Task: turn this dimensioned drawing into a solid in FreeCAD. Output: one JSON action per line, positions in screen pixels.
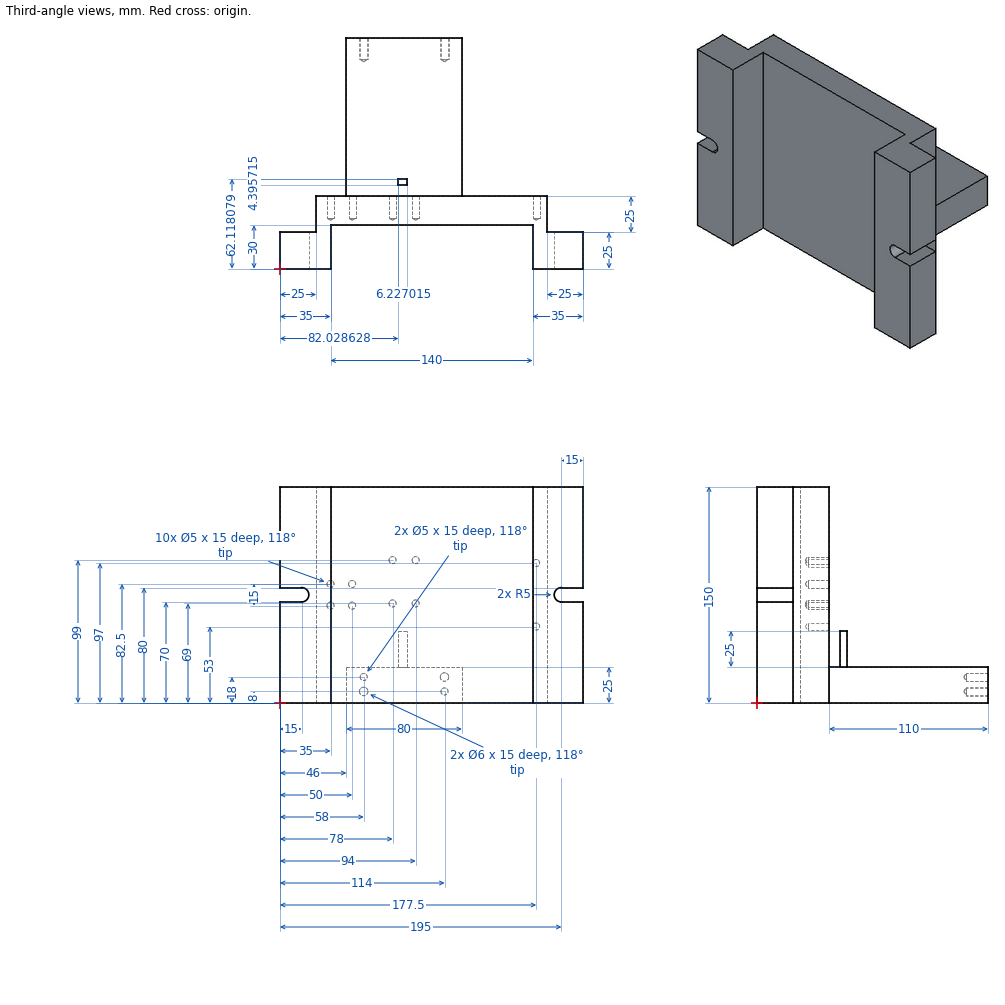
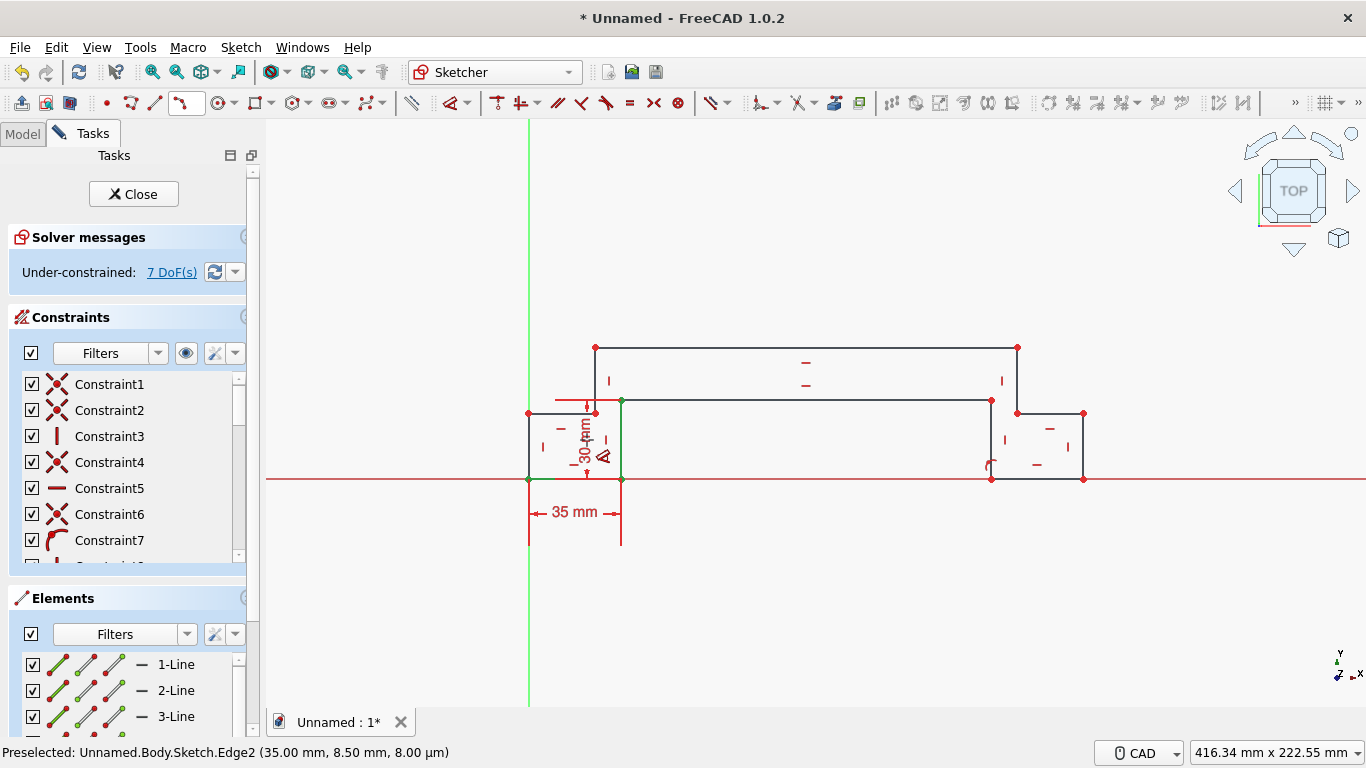
{"action": "left_click", "coordinate": [1019, 479]}
{"action": "left_click", "coordinate": [1037, 513]}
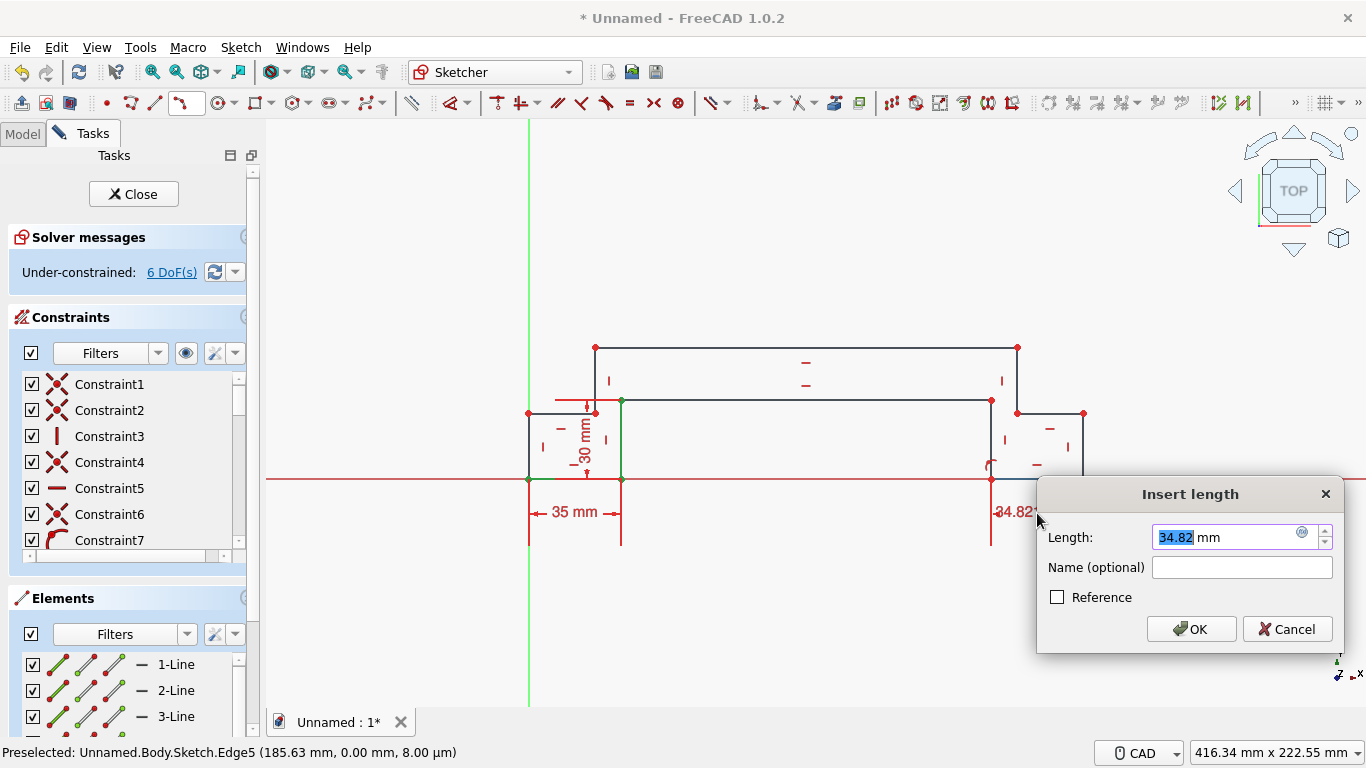
{"action": "type", "text": "35"}
{"action": "key", "text": "Return"}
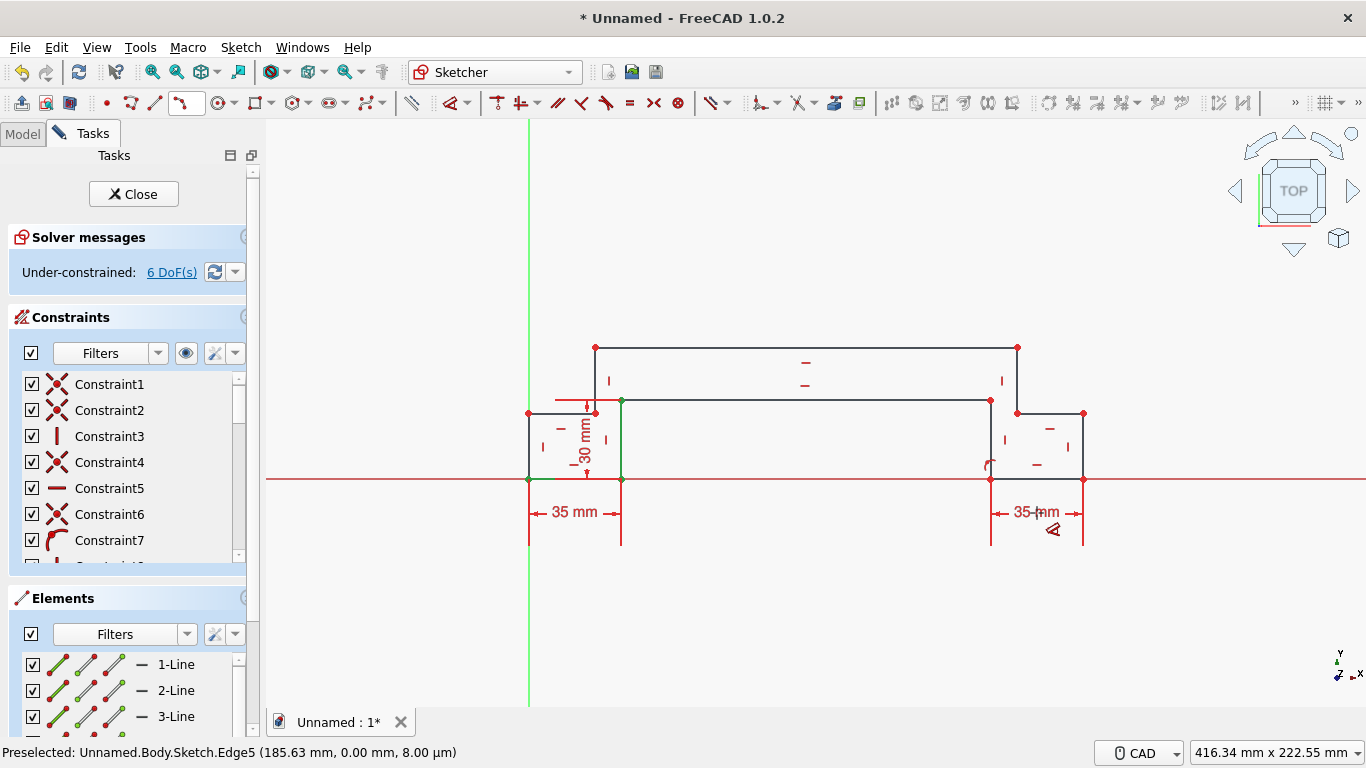
{"action": "left_click", "coordinate": [1083, 460]}
{"action": "left_click", "coordinate": [1117, 447]}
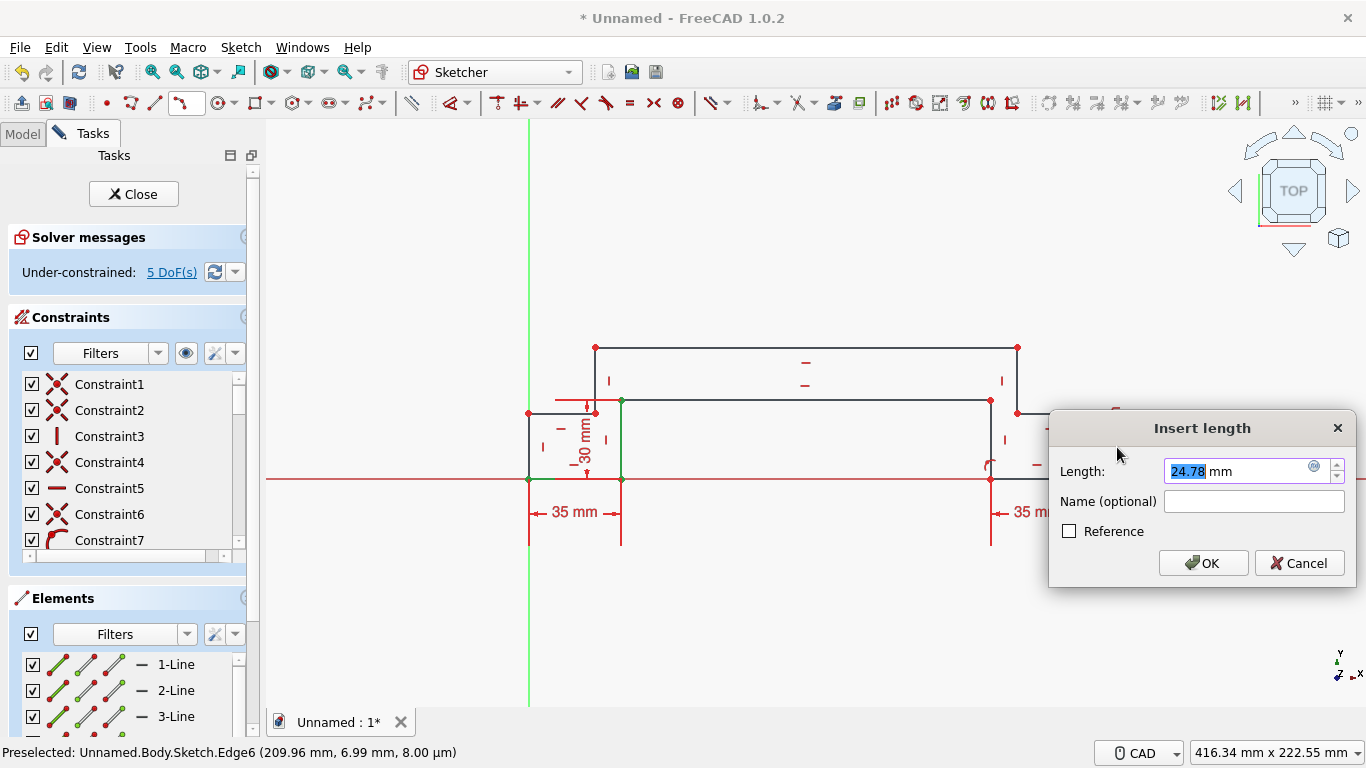
{"action": "type", "text": "25"}
{"action": "key", "text": "Return"}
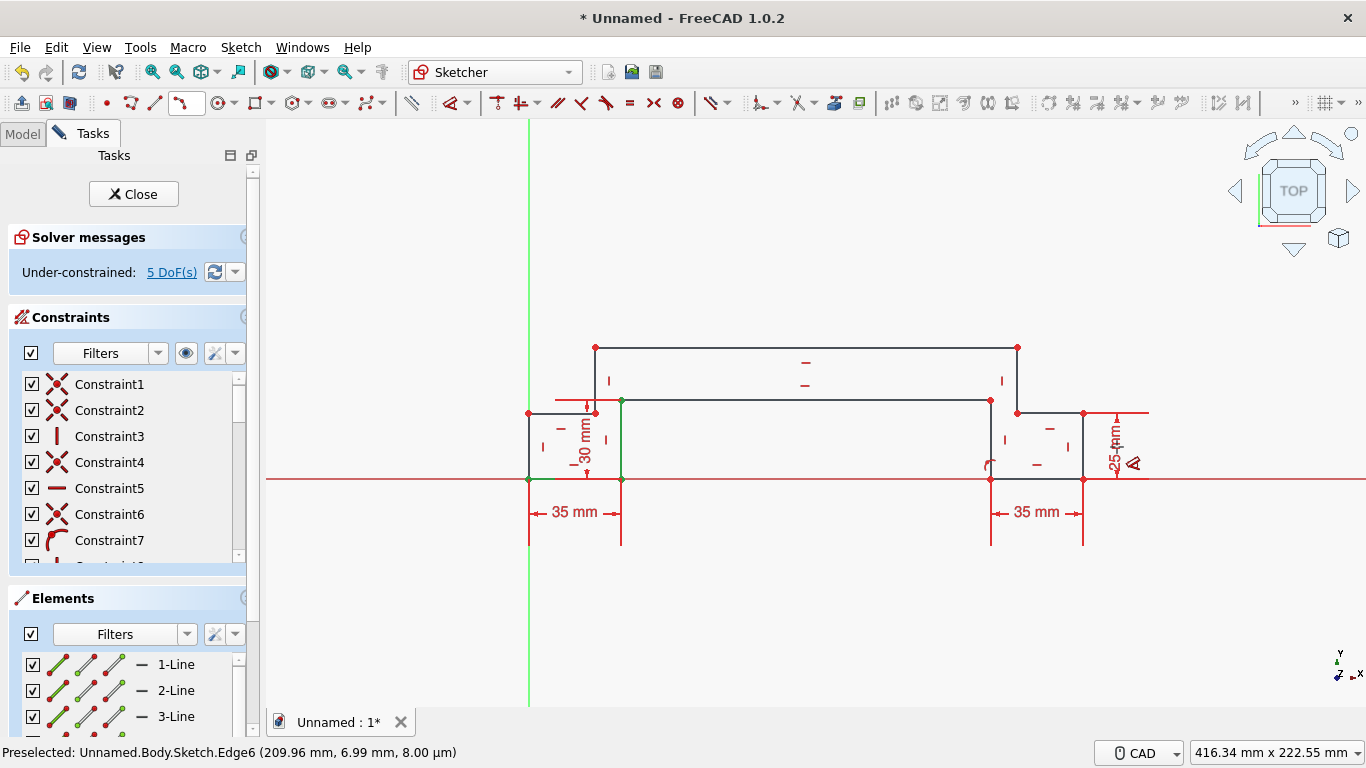
{"action": "left_click", "coordinate": [1063, 413]}
{"action": "left_click", "coordinate": [1035, 447]}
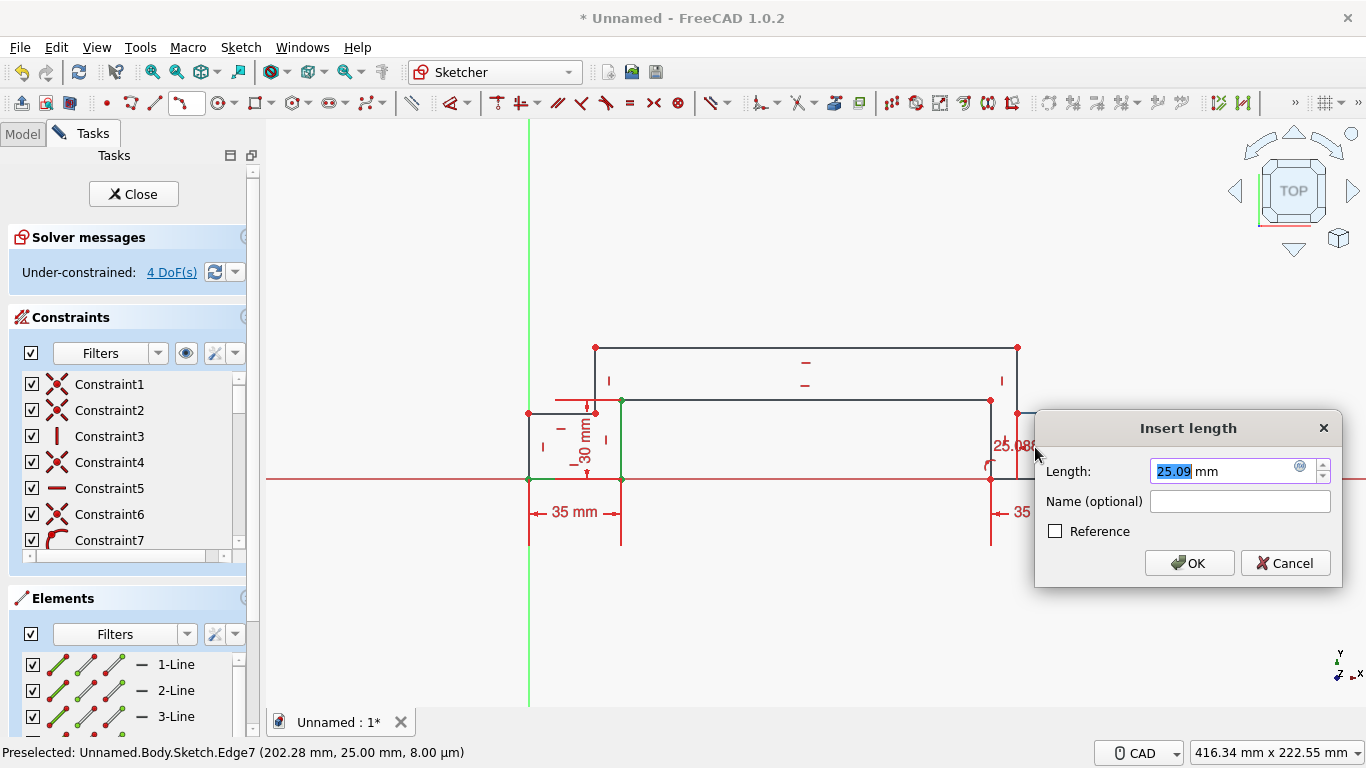
{"action": "type", "text": "25"}
{"action": "key", "text": "Return"}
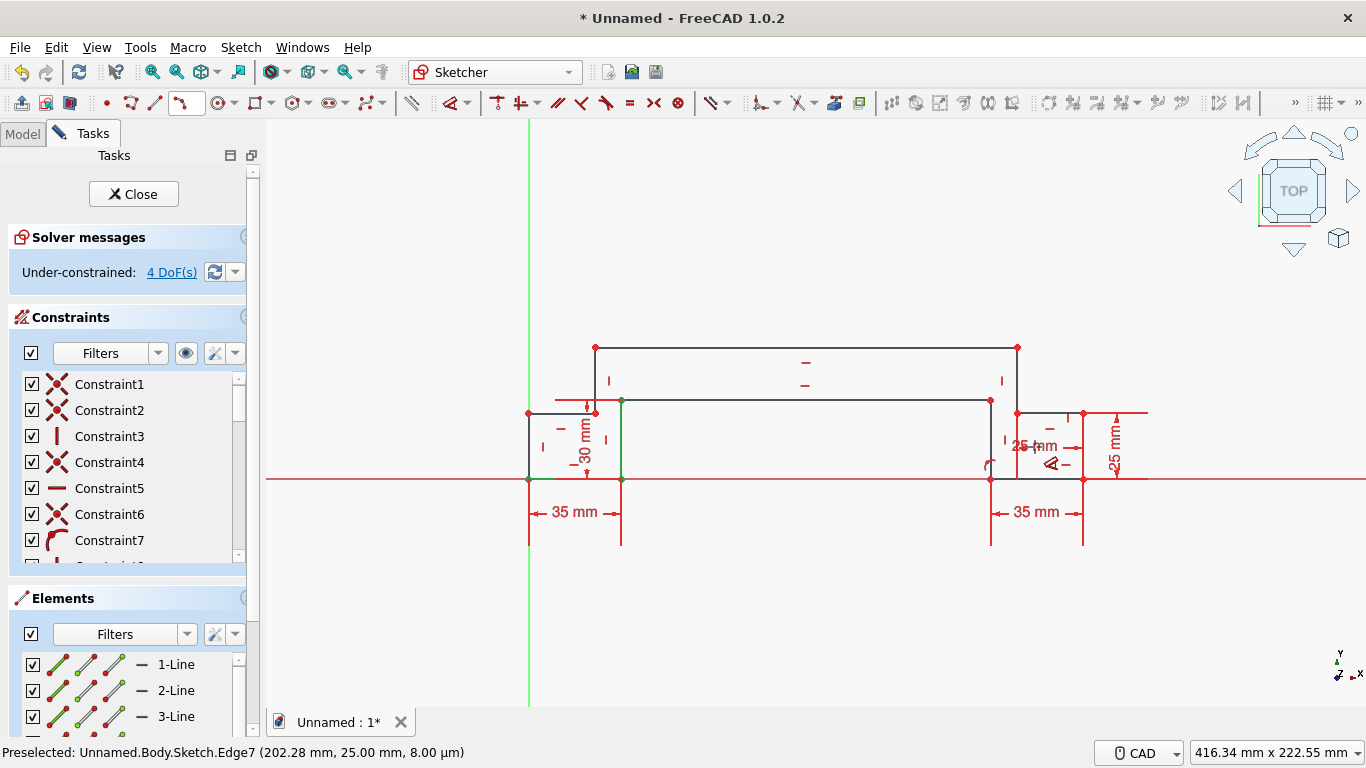
{"action": "left_click", "coordinate": [1017, 394]}
{"action": "left_click", "coordinate": [1051, 381]}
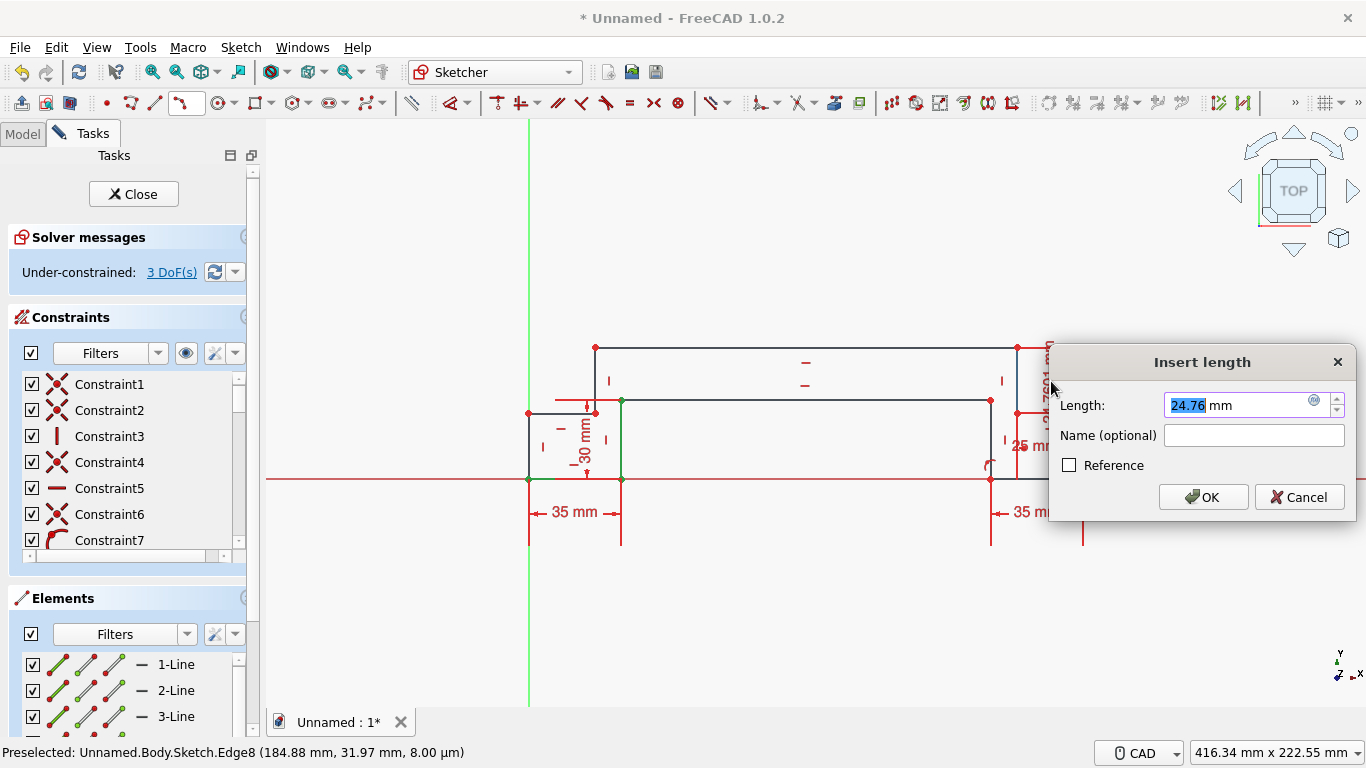
{"action": "type", "text": "25"}
{"action": "key", "text": "Return"}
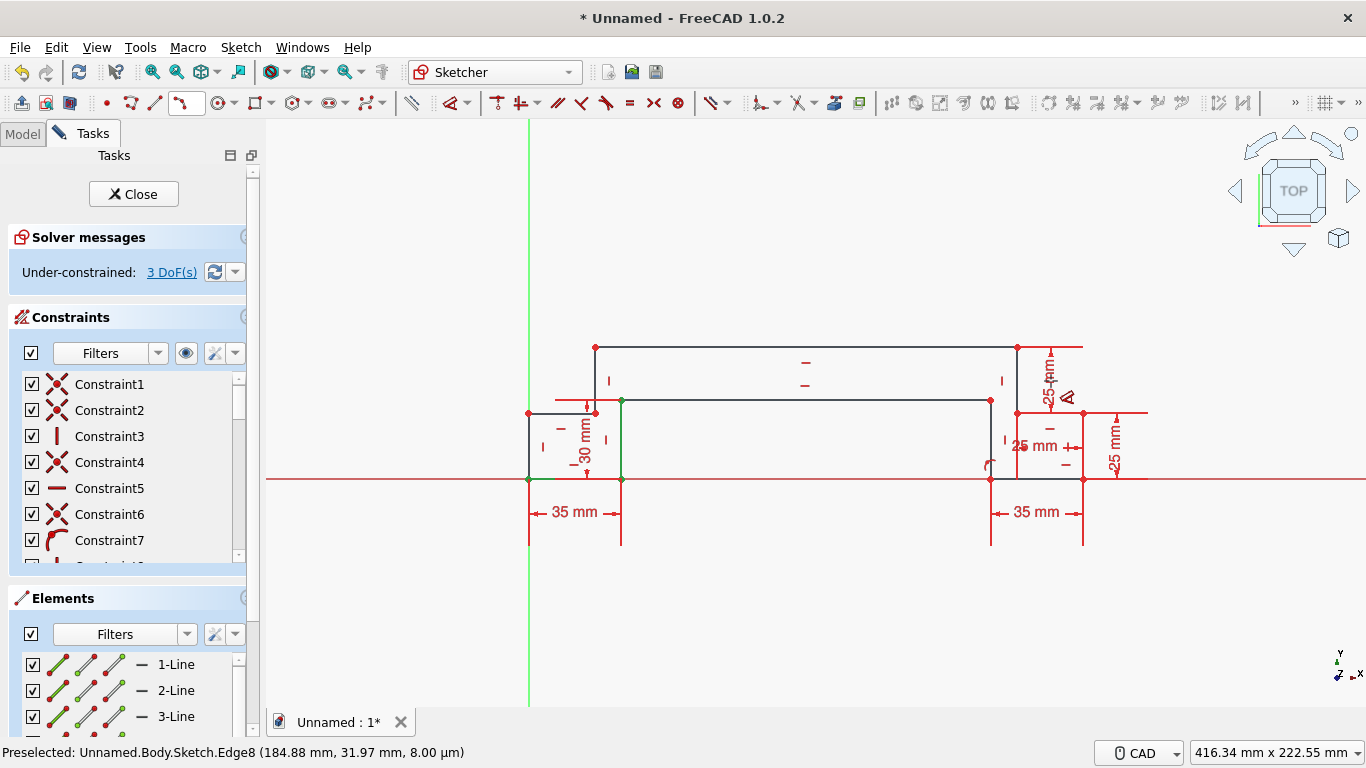
{"action": "left_click", "coordinate": [595, 367]}
{"action": "left_click", "coordinate": [561, 381]}